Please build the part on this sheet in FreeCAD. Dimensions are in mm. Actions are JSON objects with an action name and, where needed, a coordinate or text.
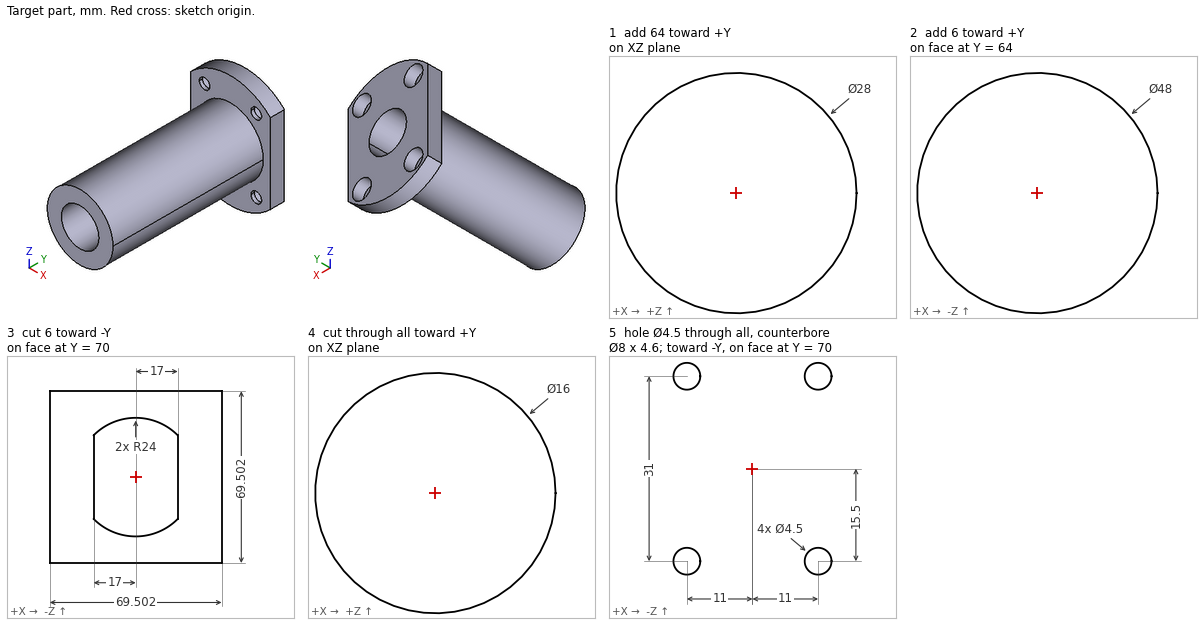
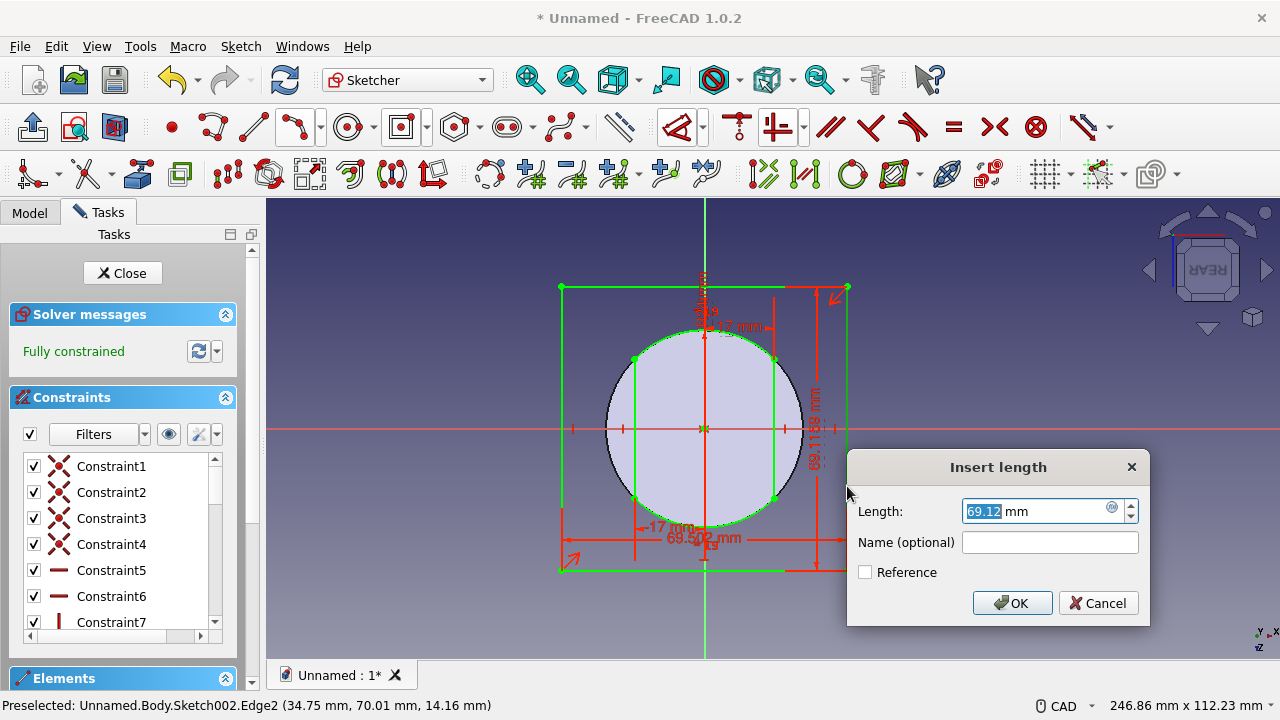
{"action": "type", "text": "69.502"}
{"action": "key", "text": "Return"}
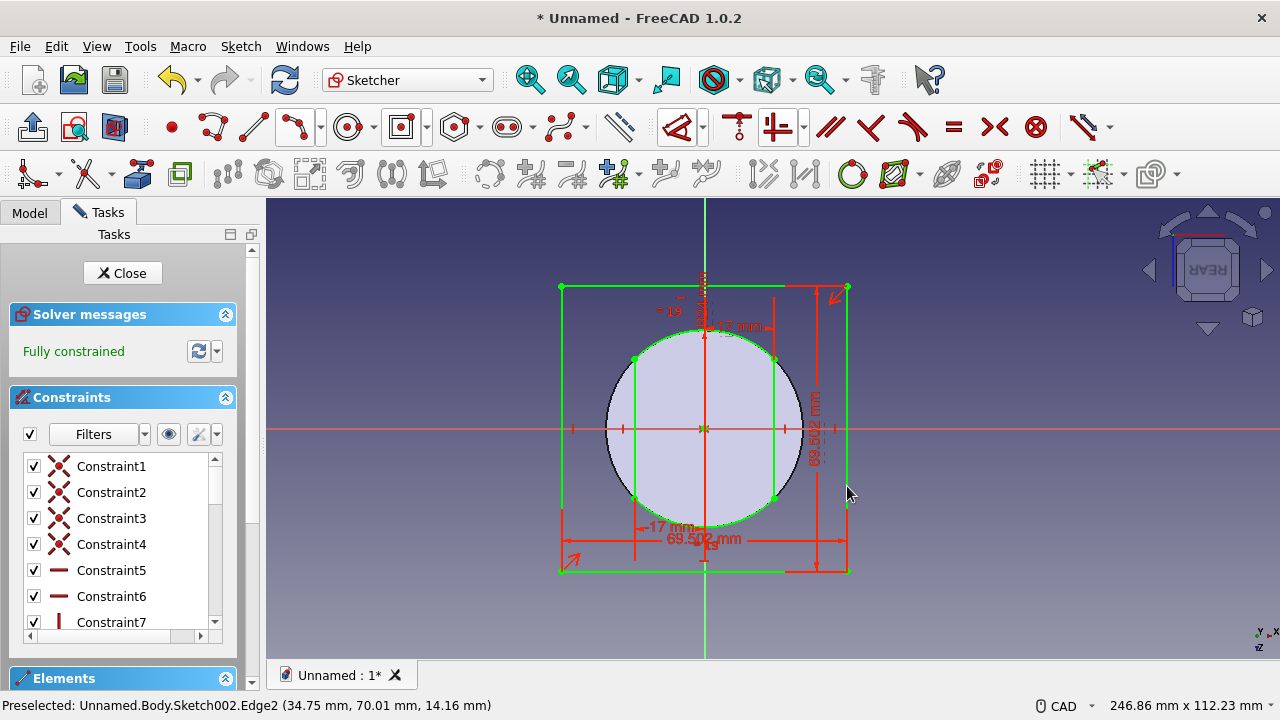
{"action": "left_click", "coordinate": [123, 273]}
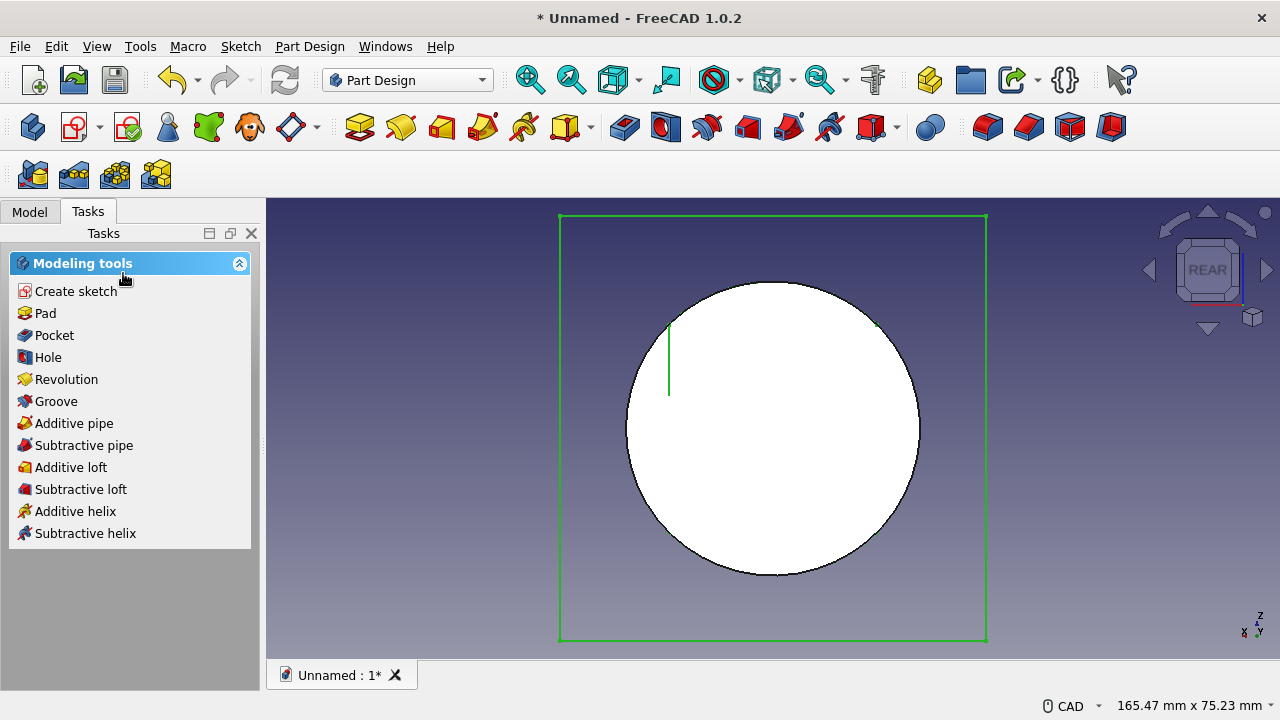
{"action": "left_click", "coordinate": [625, 128]}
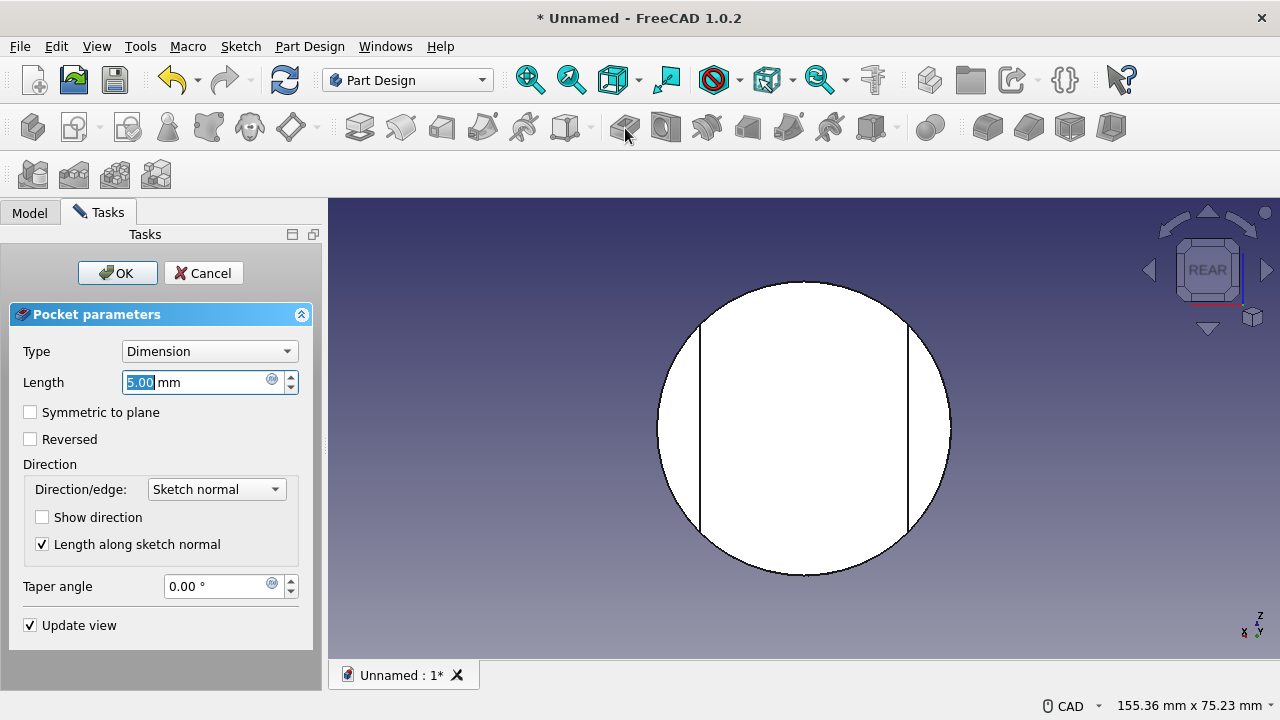
{"action": "type", "text": "6"}
{"action": "key", "text": "Tab"}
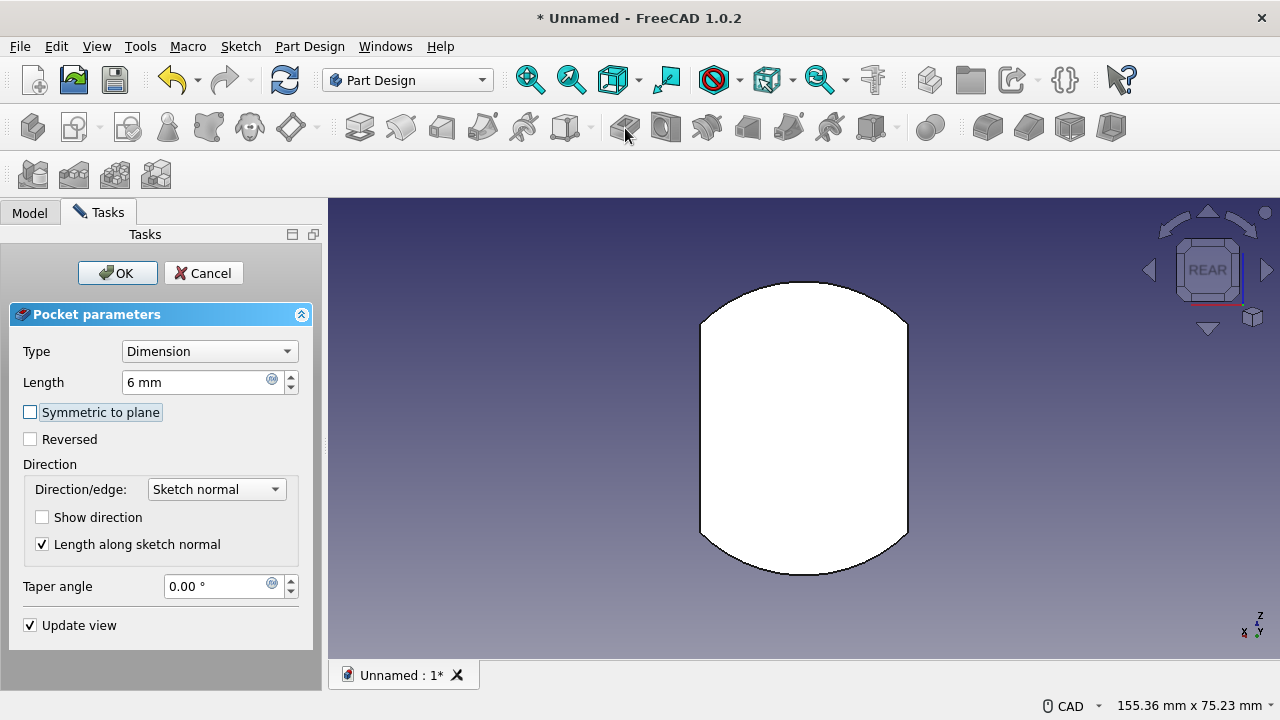
{"action": "left_click", "coordinate": [118, 273]}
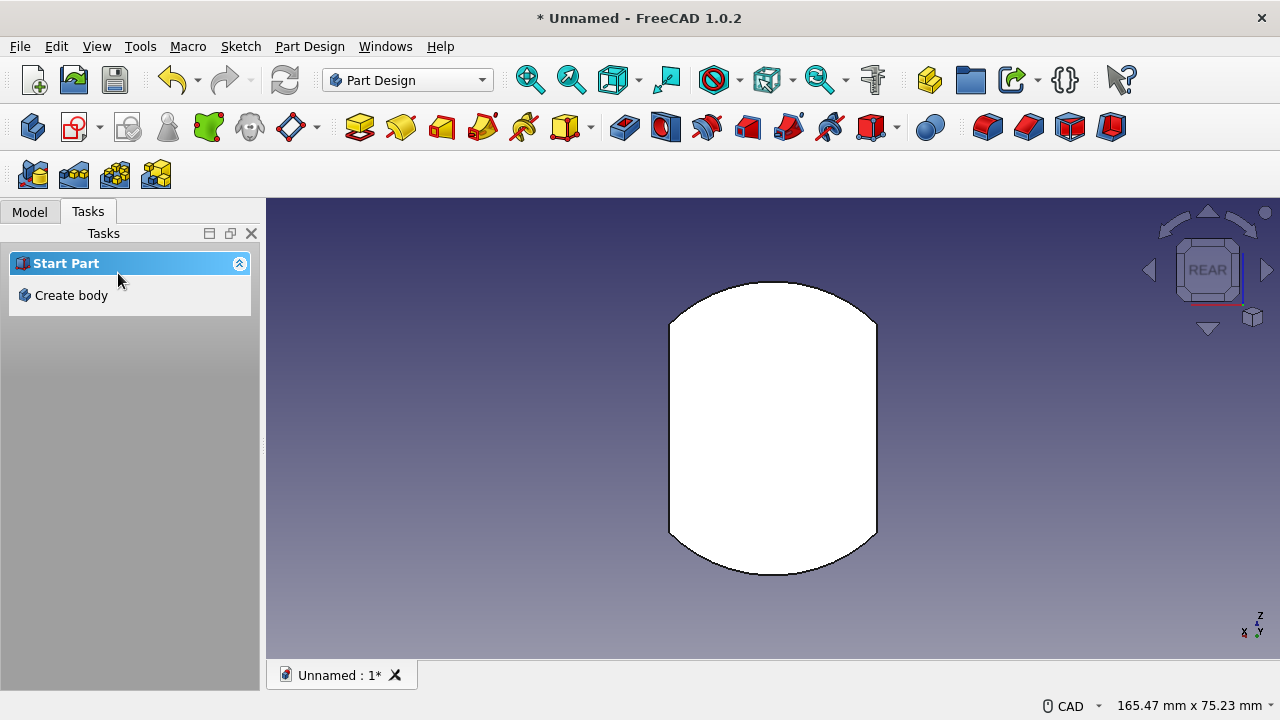
{"action": "left_click", "coordinate": [74, 128]}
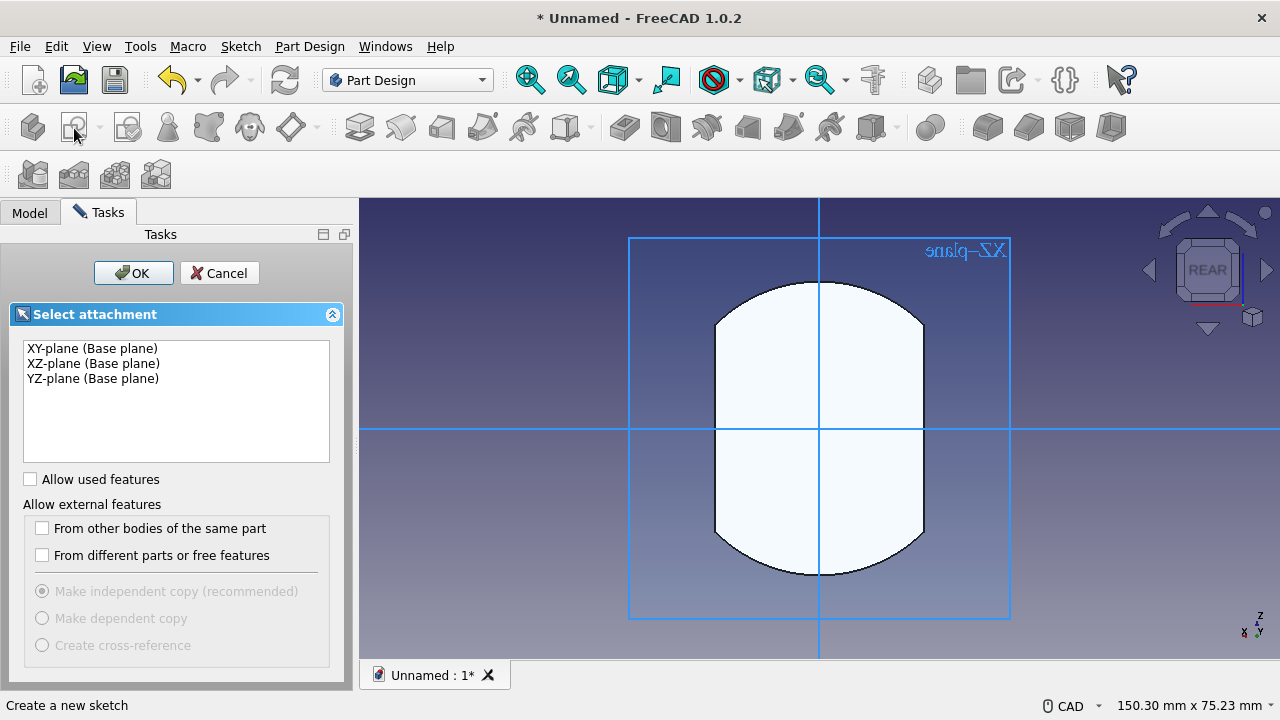
{"action": "left_click", "coordinate": [84, 364]}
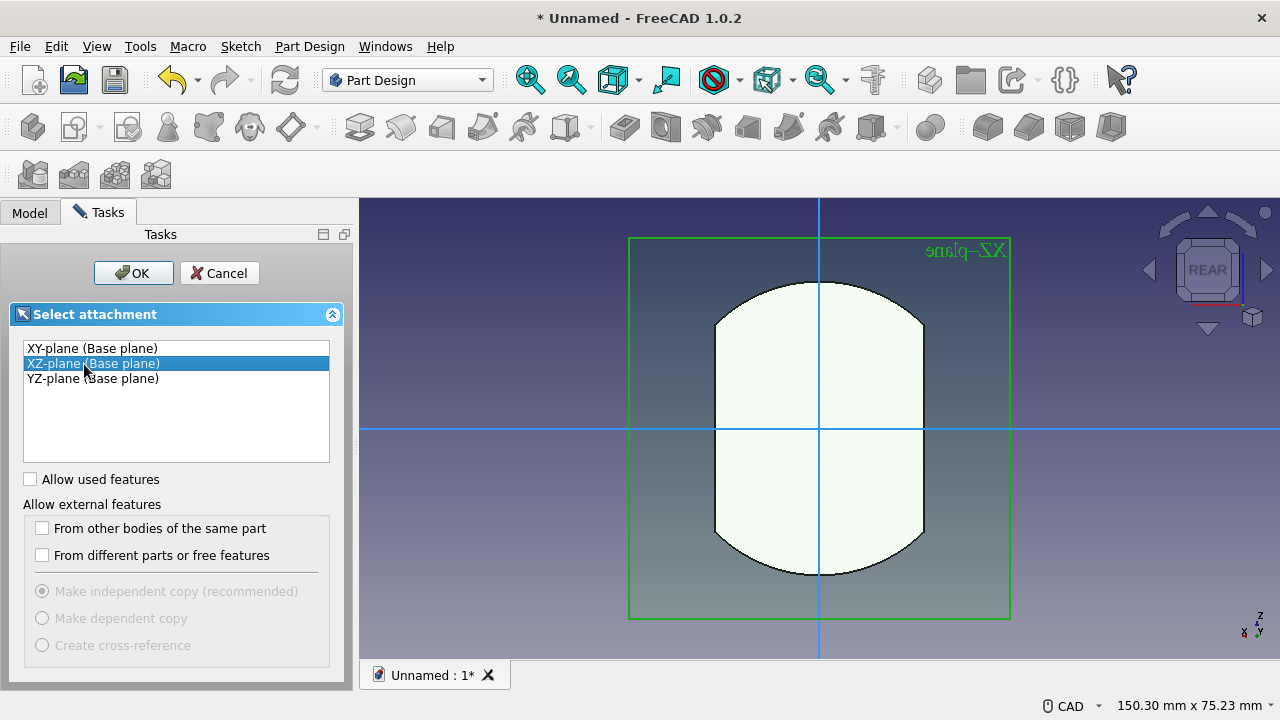
{"action": "left_click", "coordinate": [134, 273]}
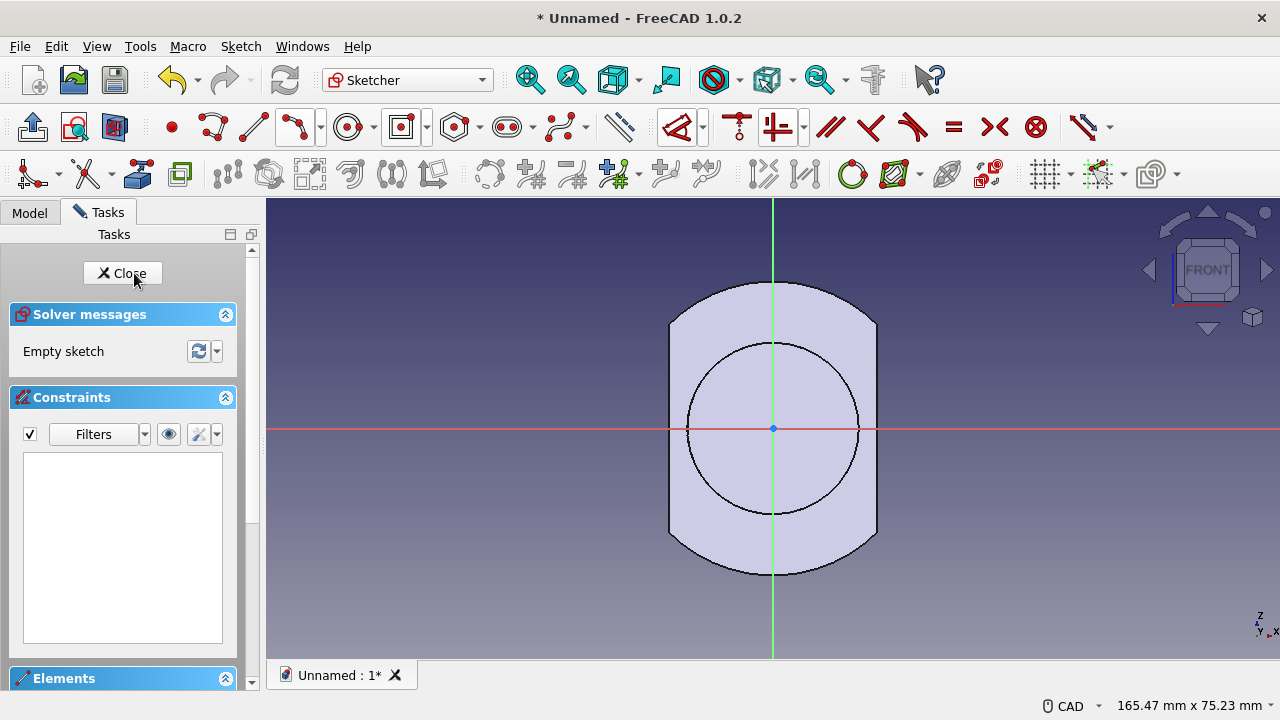
{"action": "scroll", "coordinate": [813, 429], "scroll_direction": "up", "scroll_amount": 5}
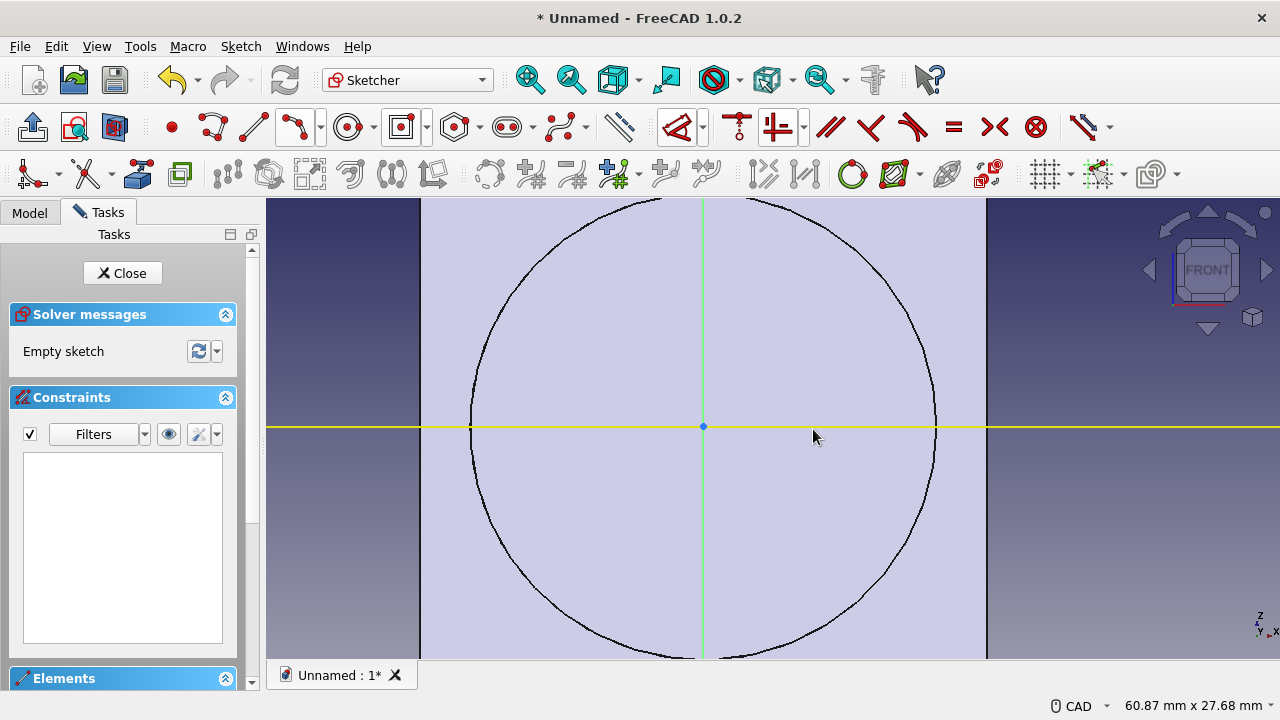
{"action": "left_click", "coordinate": [348, 128]}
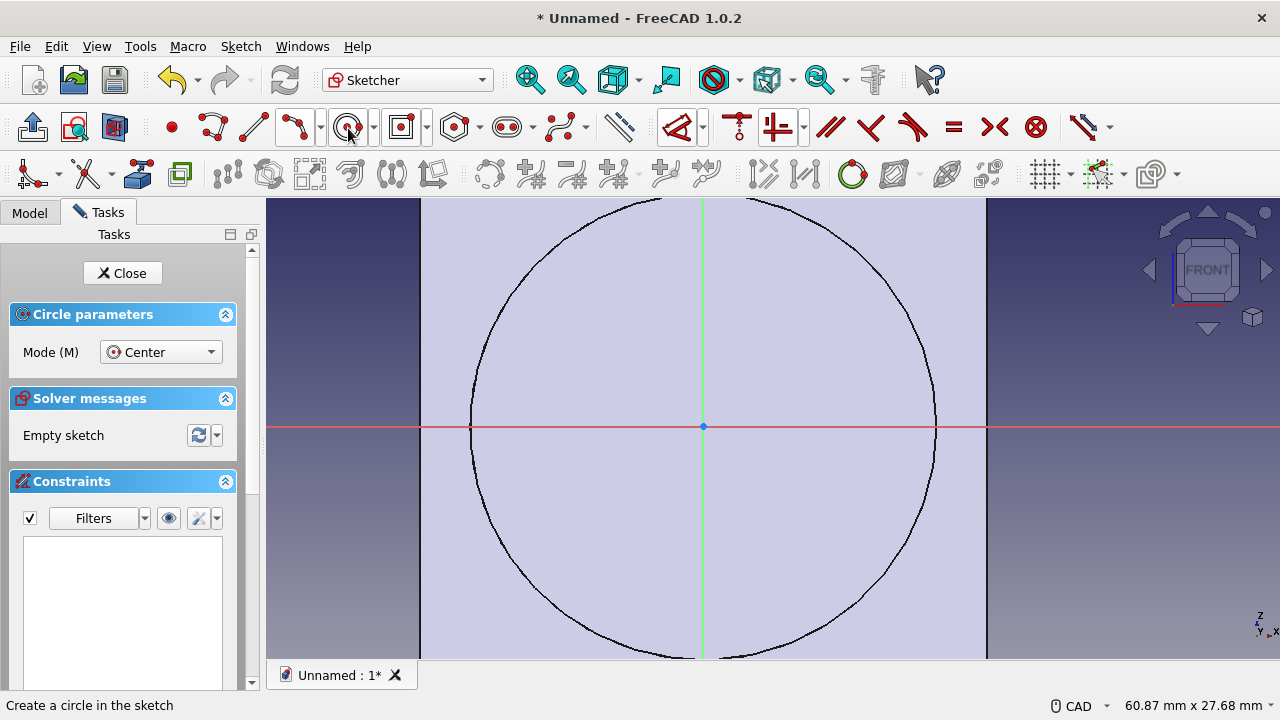
{"action": "left_click", "coordinate": [703, 427]}
{"action": "left_click", "coordinate": [798, 333]}
{"action": "key", "text": "Escape"}